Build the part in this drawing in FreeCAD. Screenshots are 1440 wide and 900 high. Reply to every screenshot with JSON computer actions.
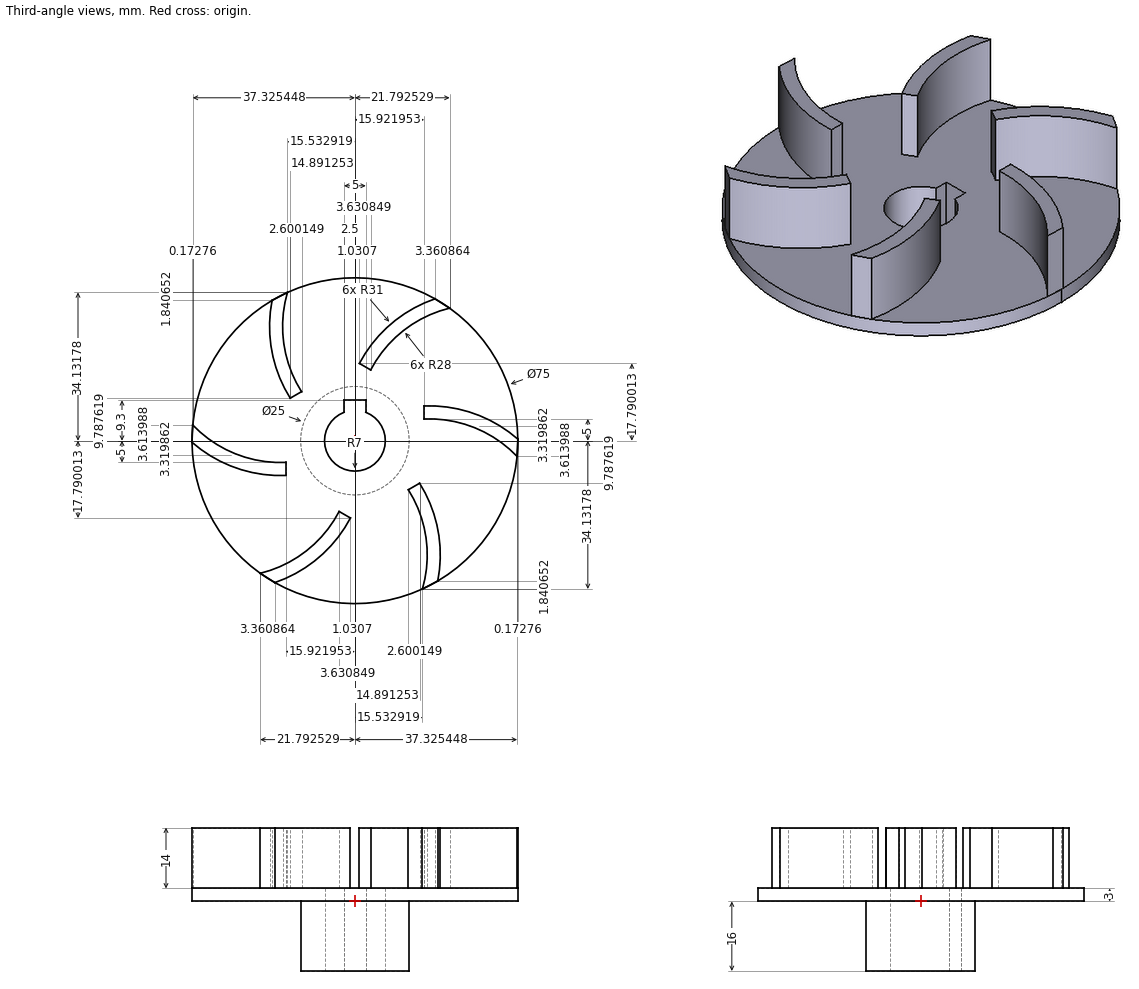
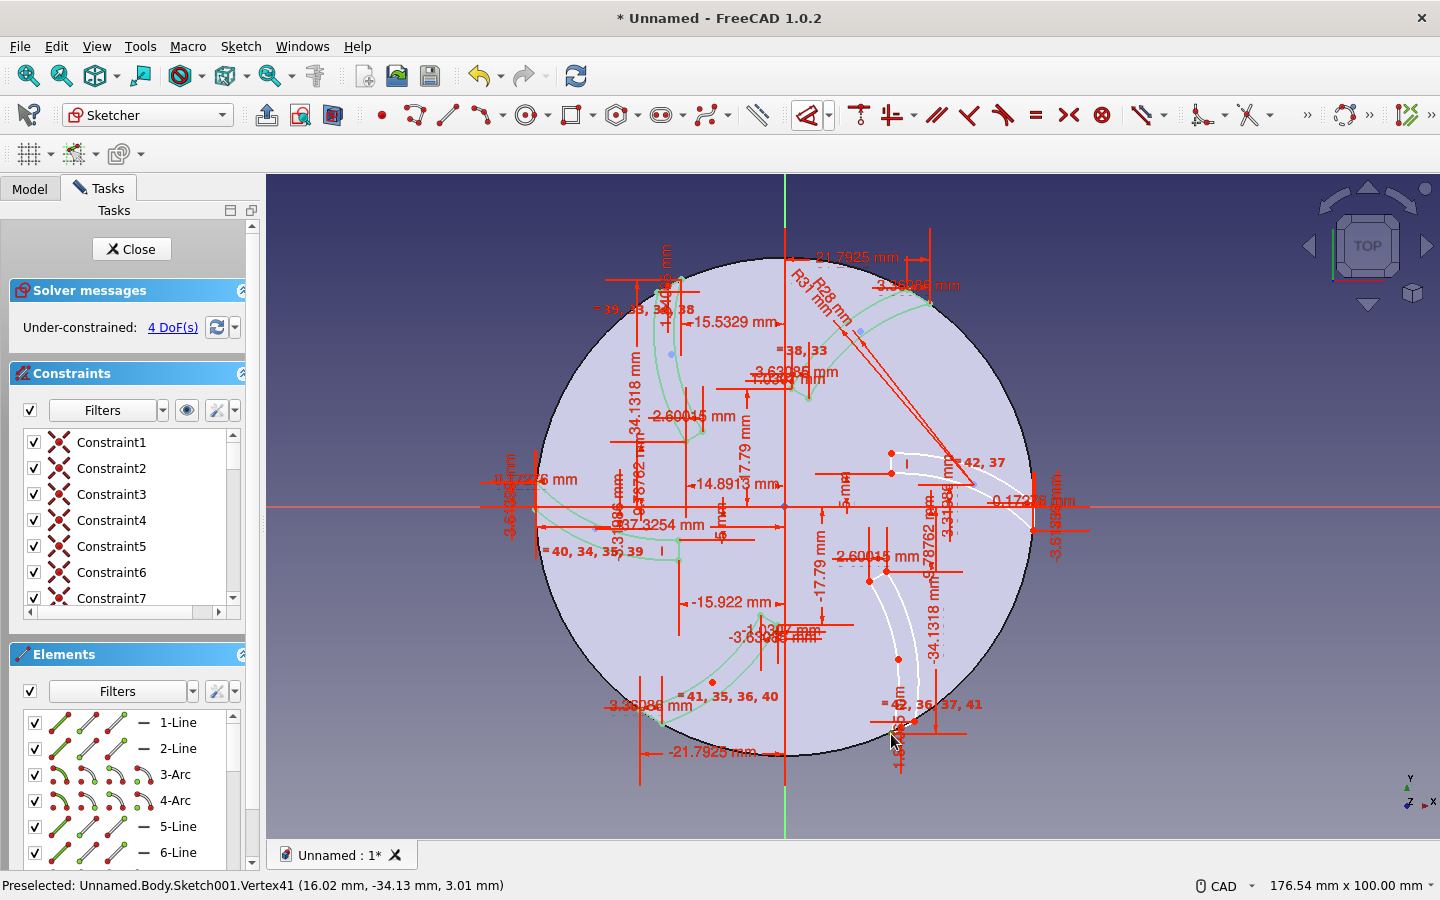
{"action": "left_click", "coordinate": [828, 116]}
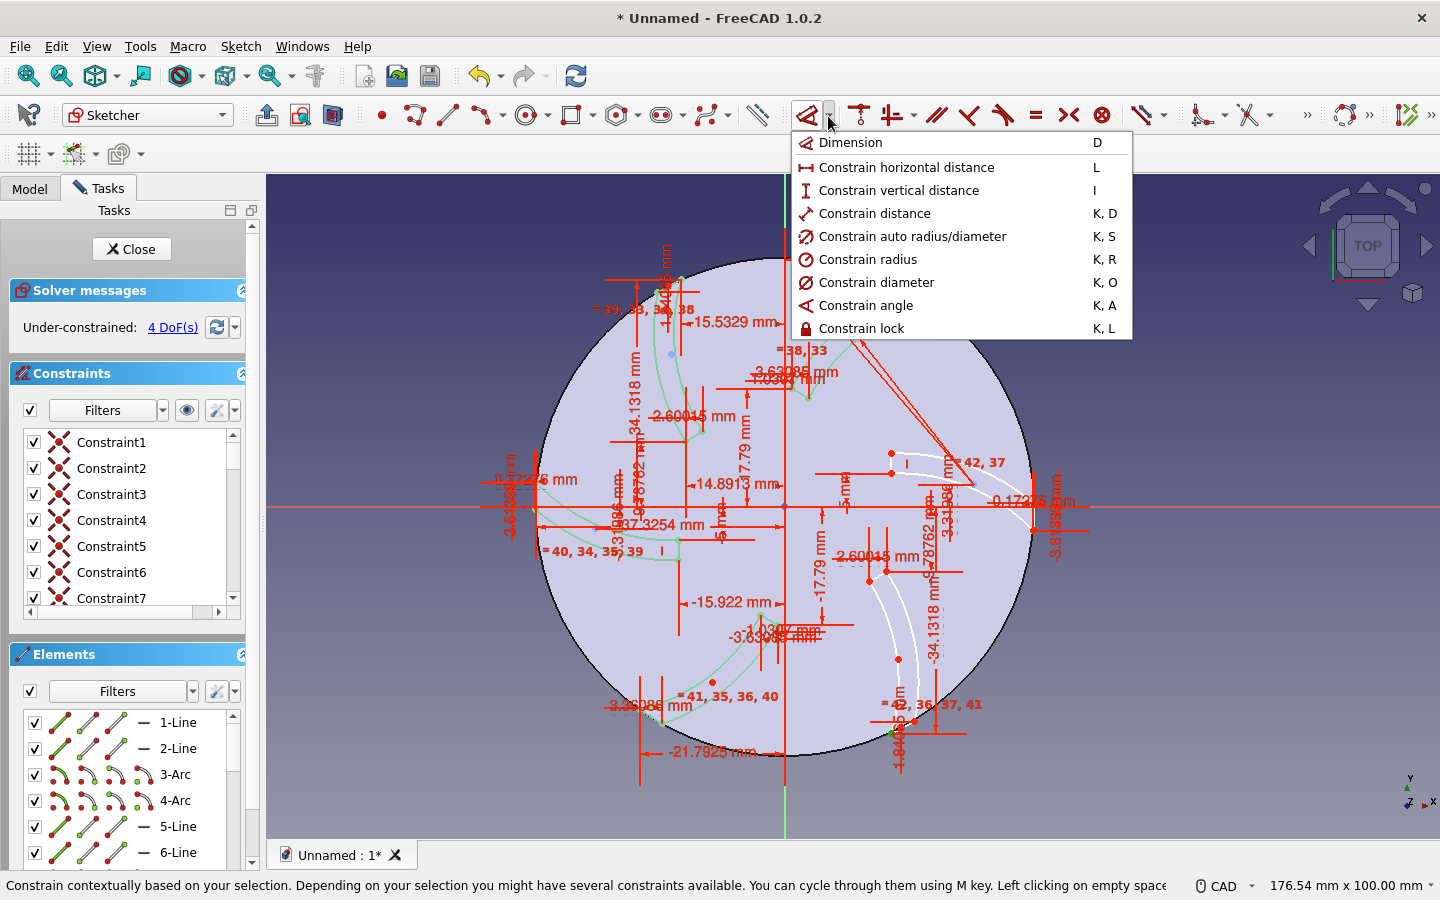
{"action": "left_click", "coordinate": [962, 168]}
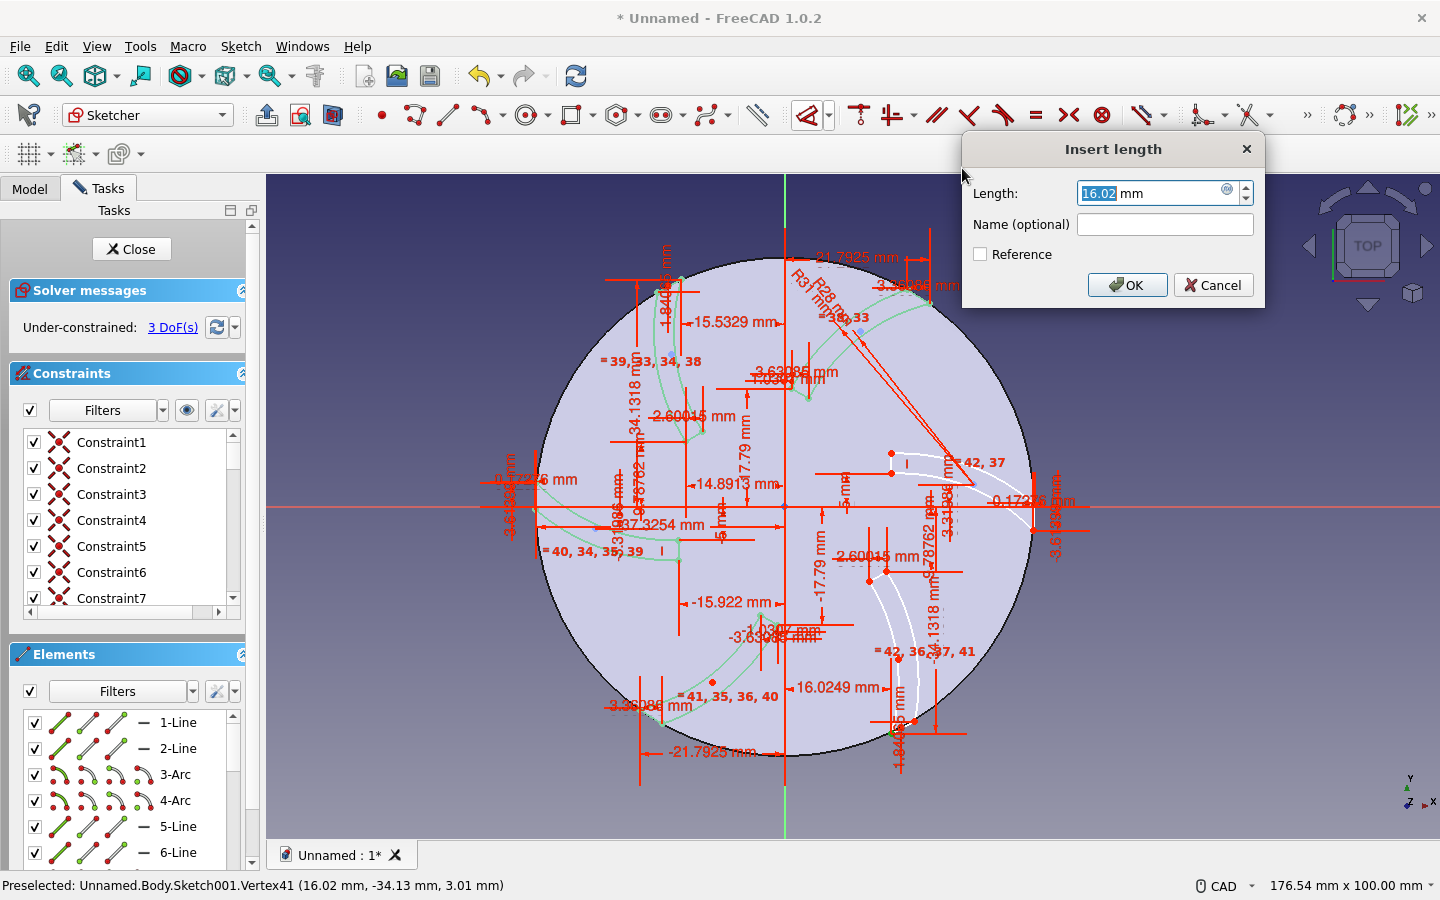
{"action": "type", "text": "15.532919"}
{"action": "key", "text": "Return"}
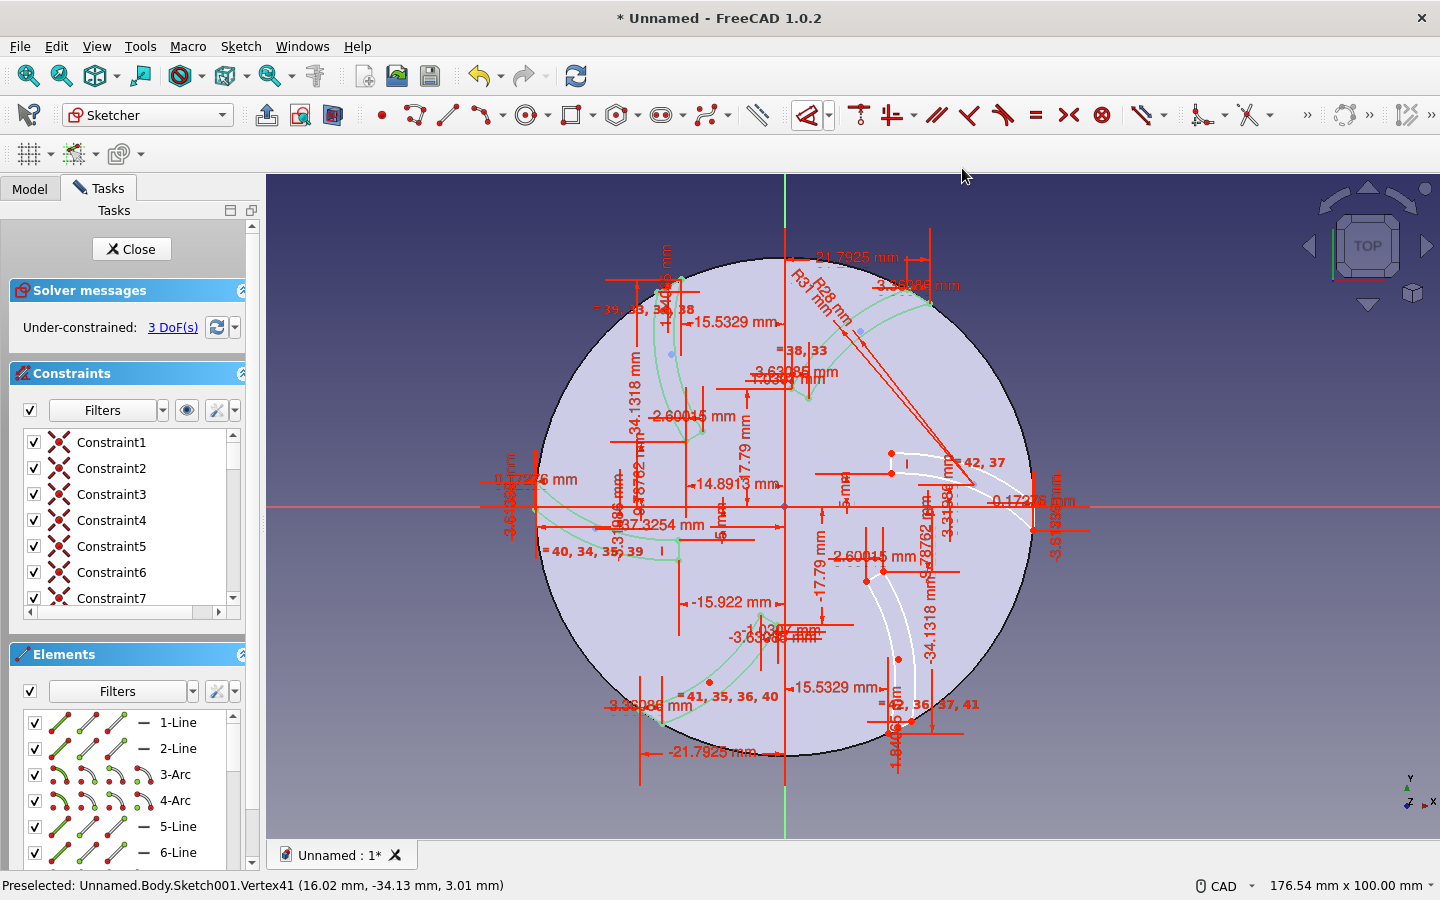
{"action": "left_click", "coordinate": [883, 572]}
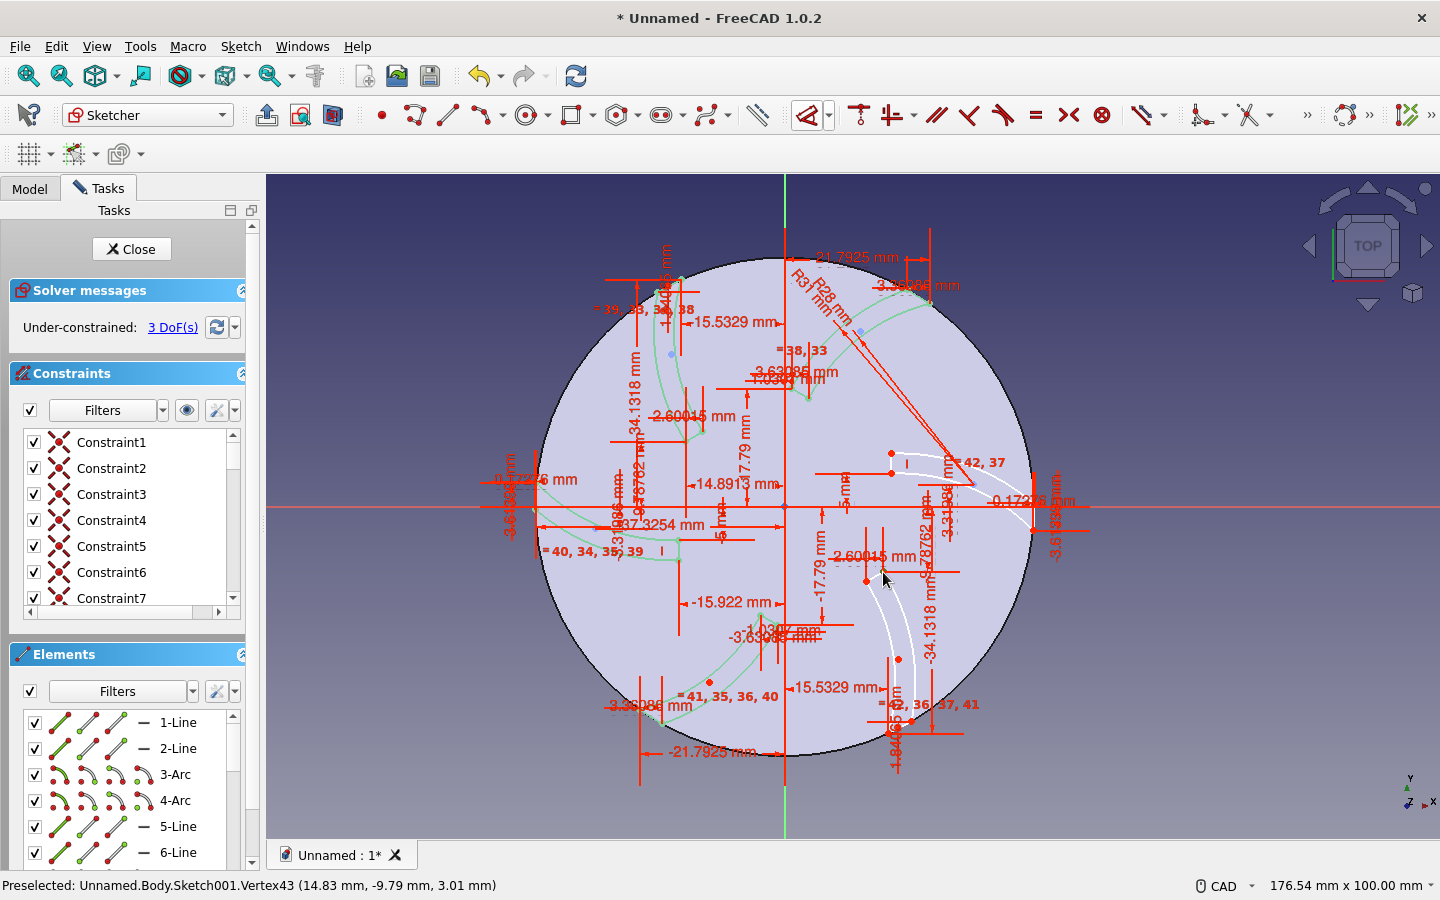
{"action": "key", "text": "l"}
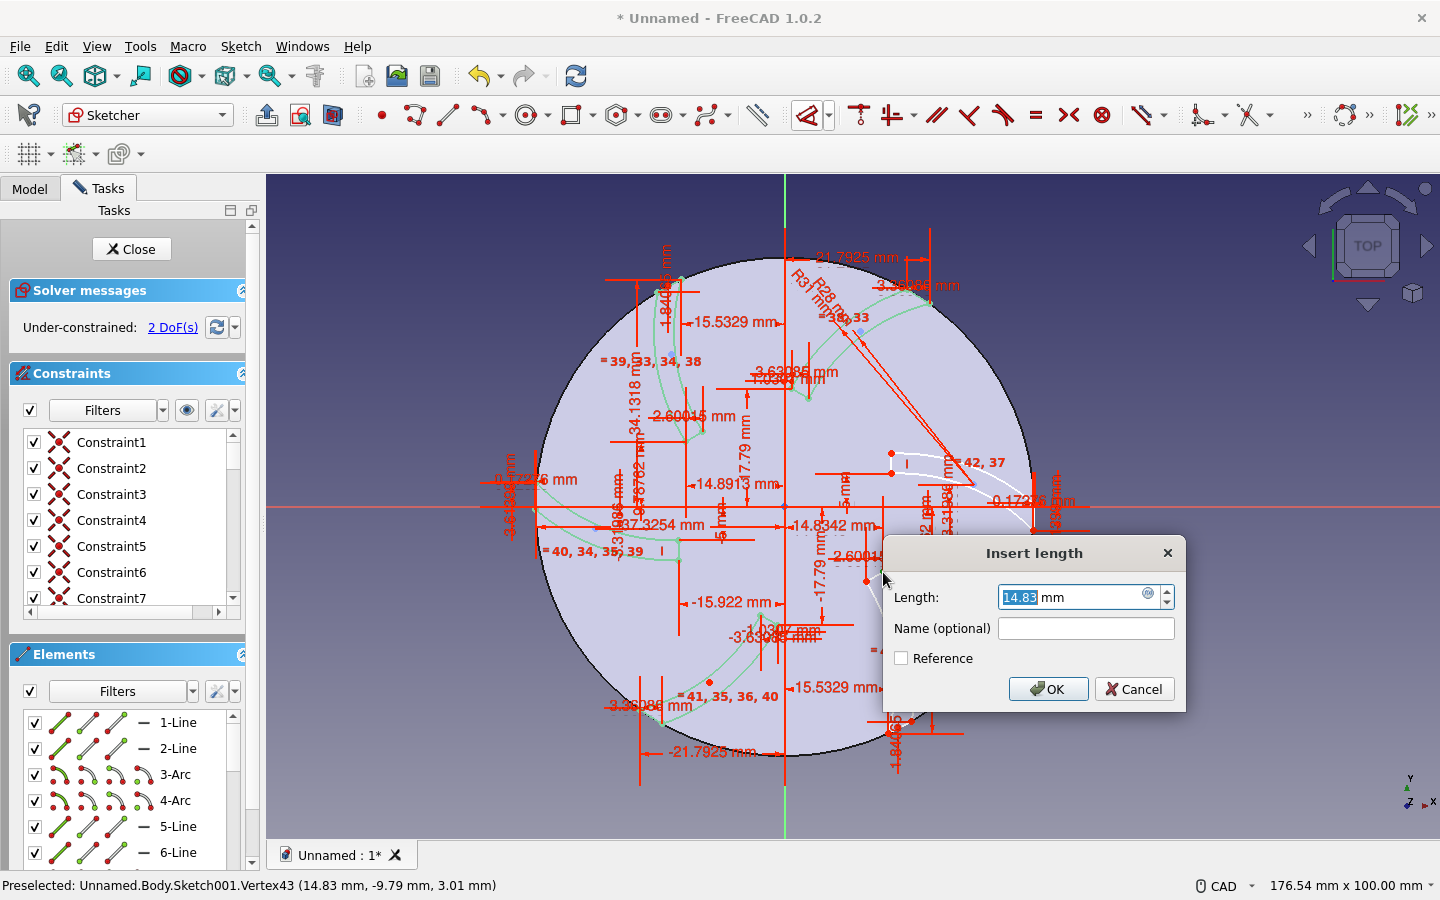
{"action": "type", "text": "14.891253"}
{"action": "key", "text": "Return"}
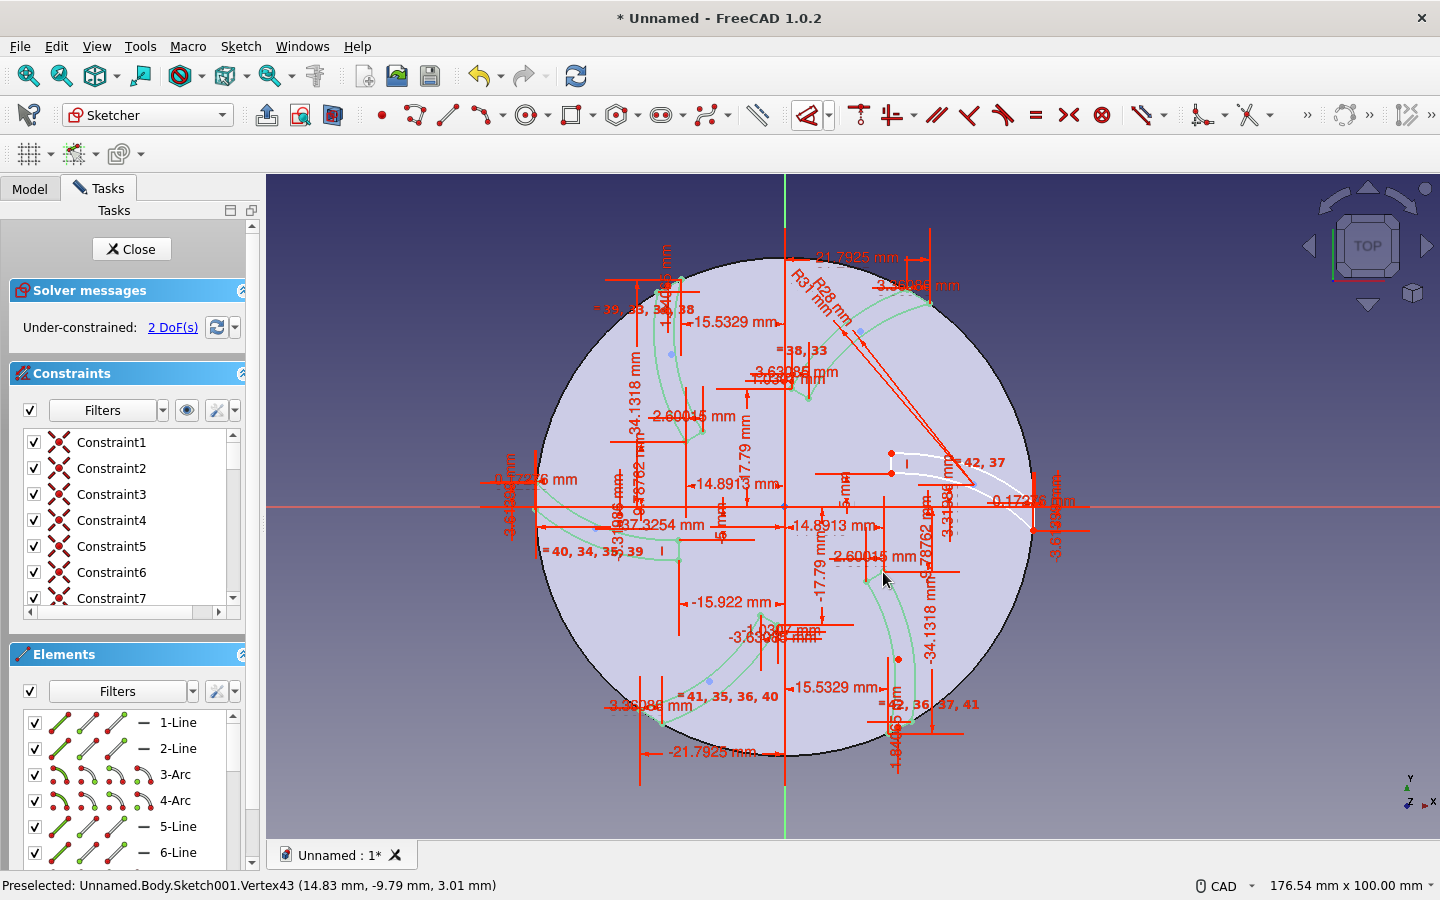
{"action": "left_click", "coordinate": [1033, 531]}